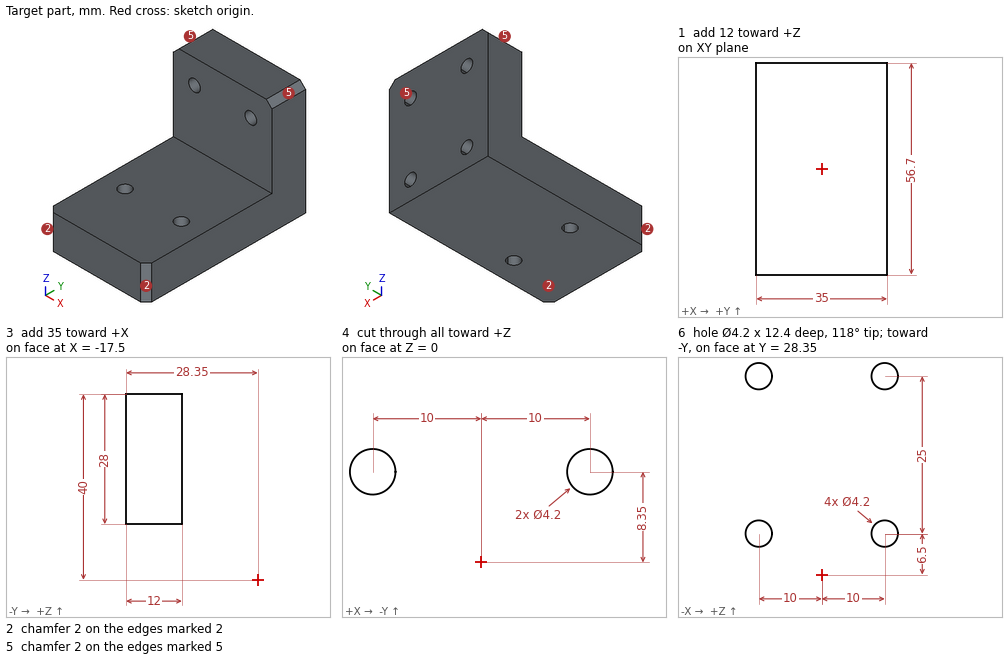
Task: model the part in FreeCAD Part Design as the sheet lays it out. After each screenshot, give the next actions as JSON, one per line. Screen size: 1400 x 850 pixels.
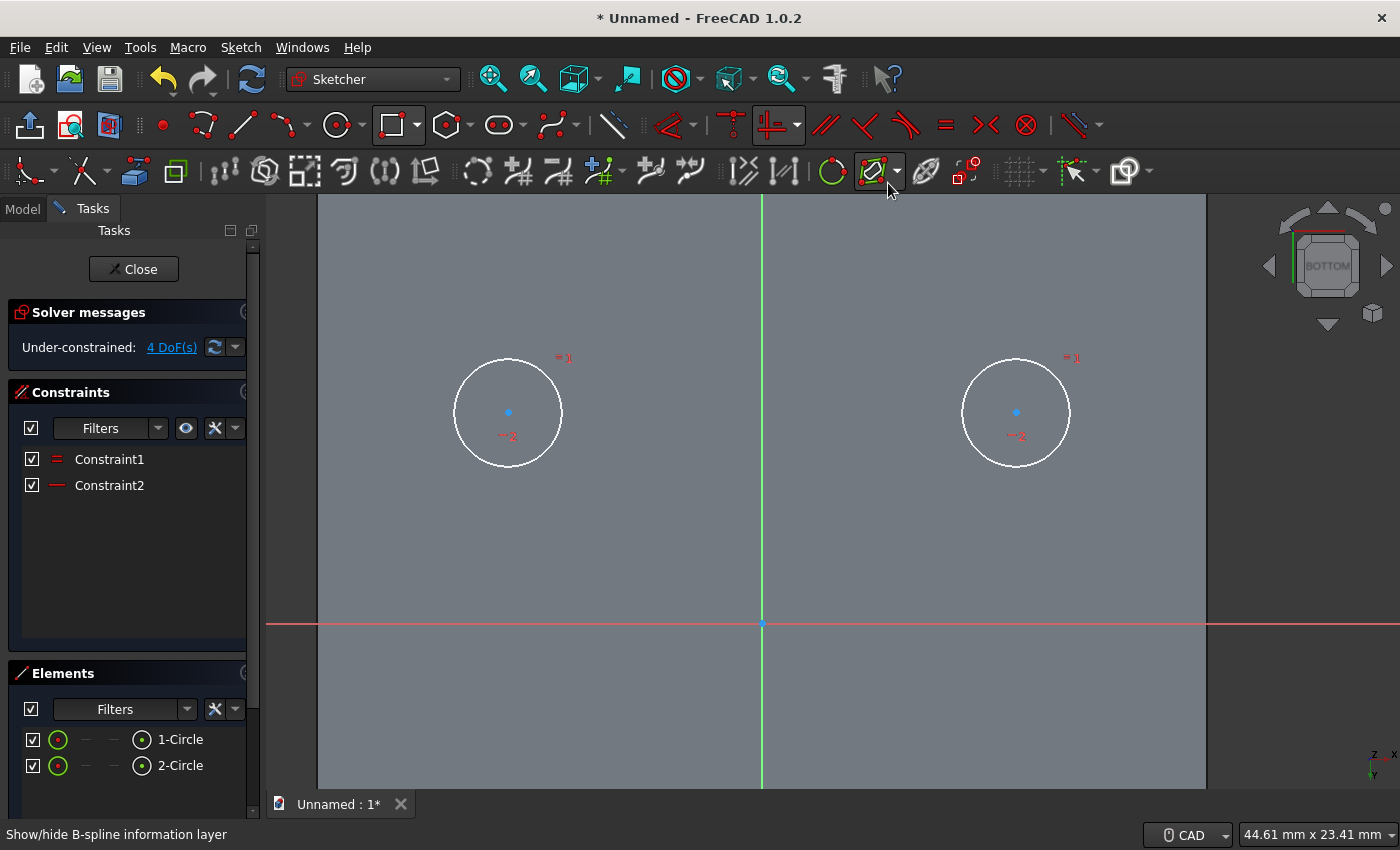
{"action": "left_click", "coordinate": [668, 126]}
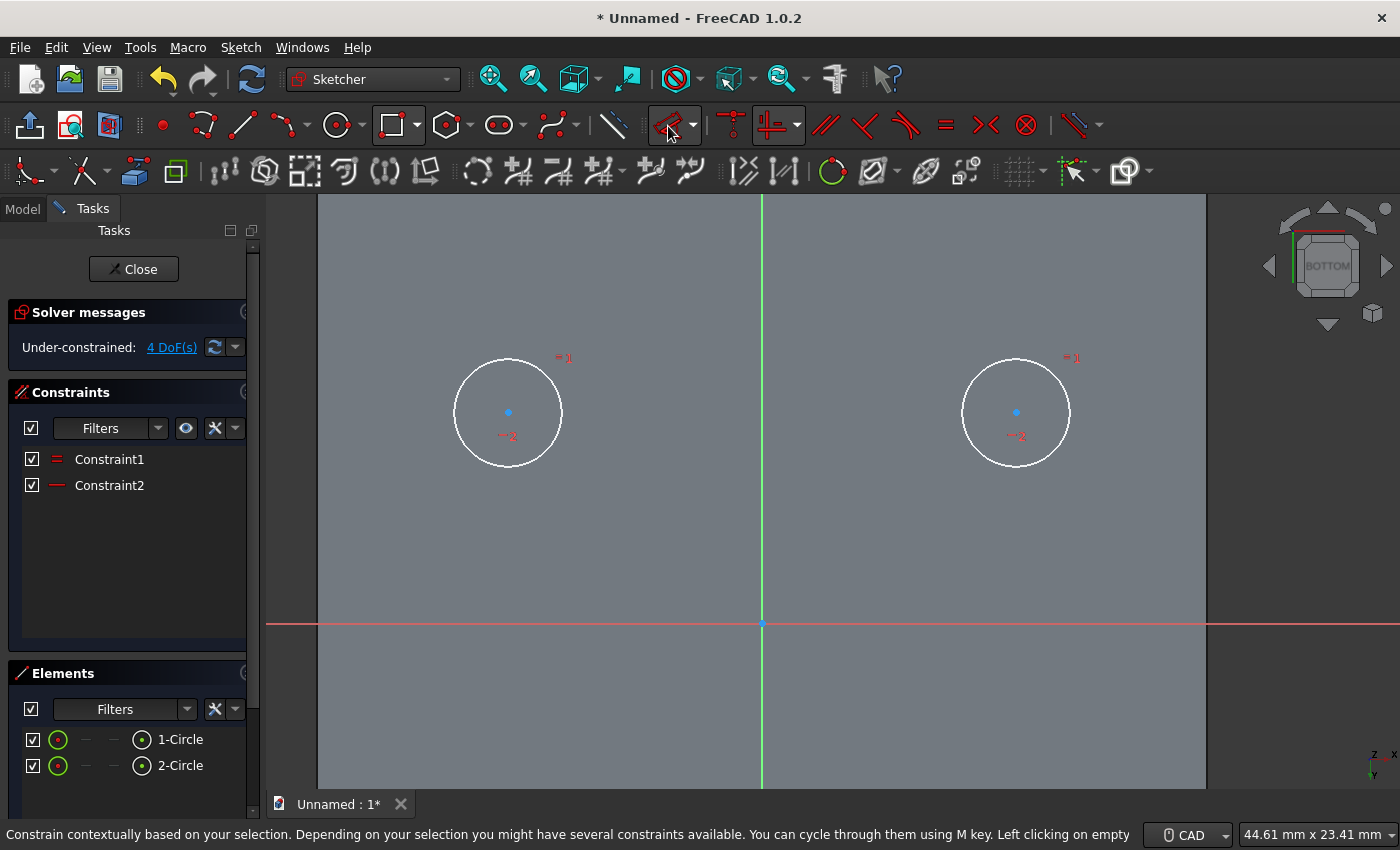
{"action": "left_click", "coordinate": [1054, 375]}
{"action": "left_click", "coordinate": [1077, 352]}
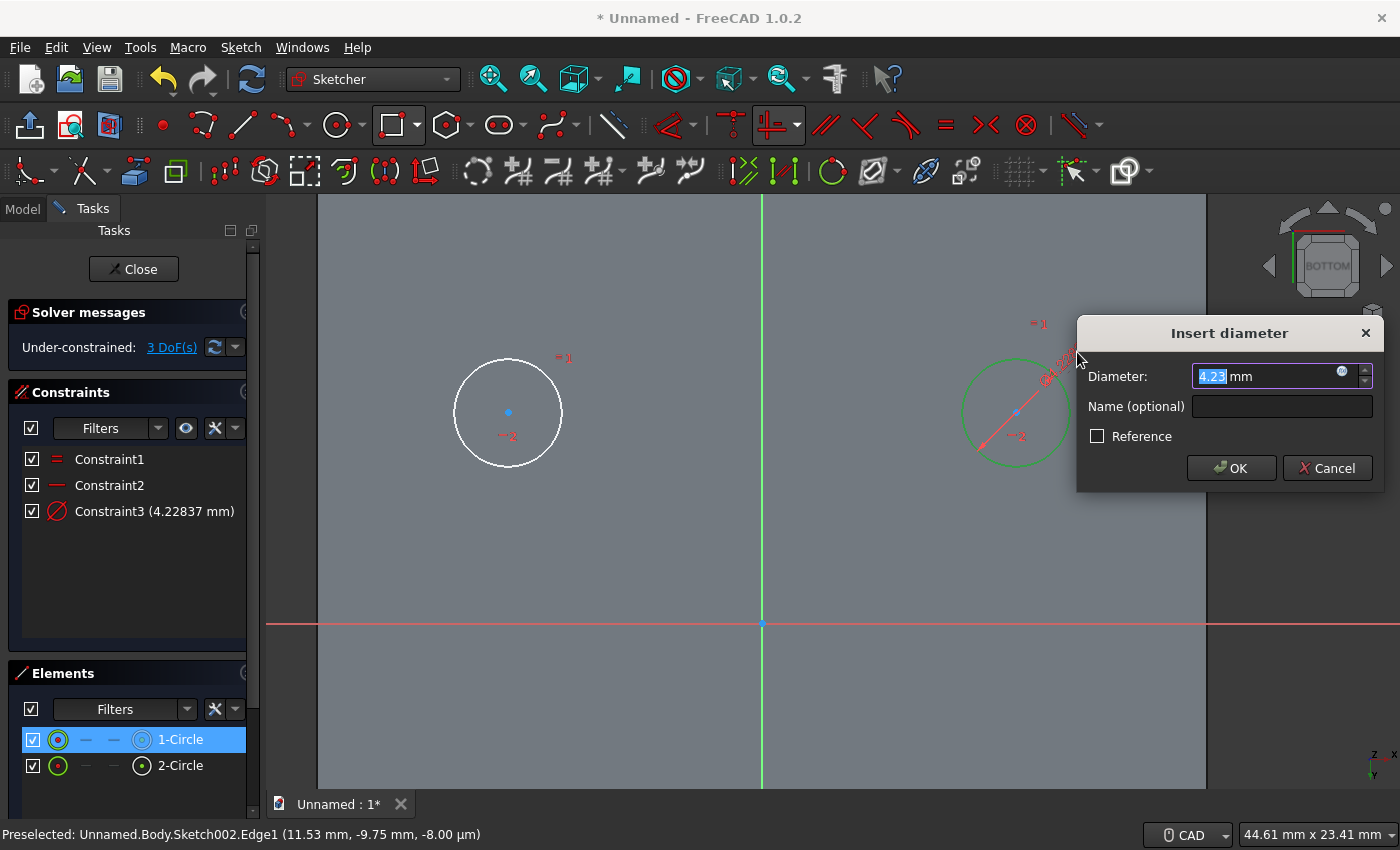
{"action": "type", "text": "4.2"}
{"action": "key", "text": "Return"}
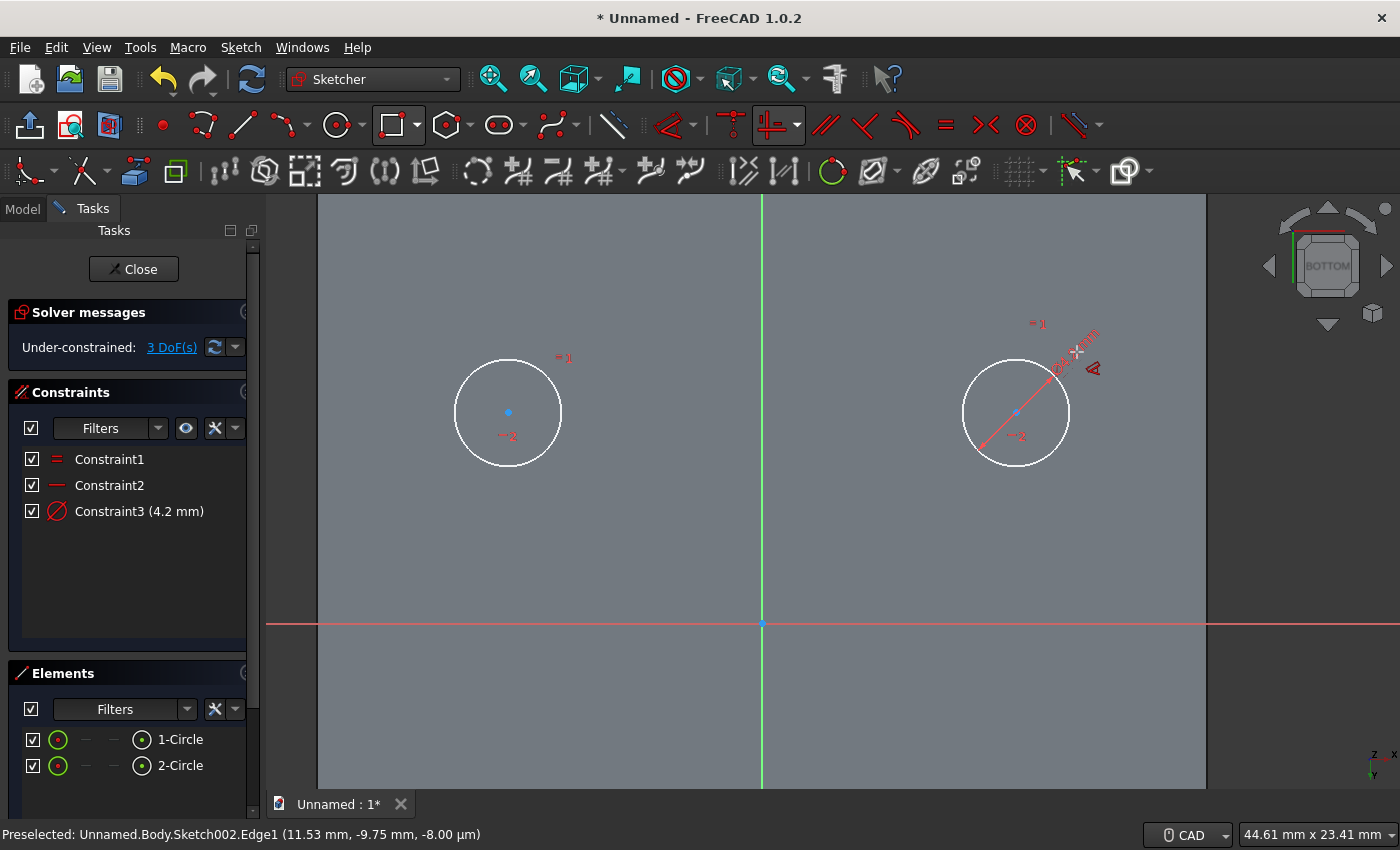
{"action": "left_click", "coordinate": [1016, 413]}
{"action": "left_click", "coordinate": [889, 658]}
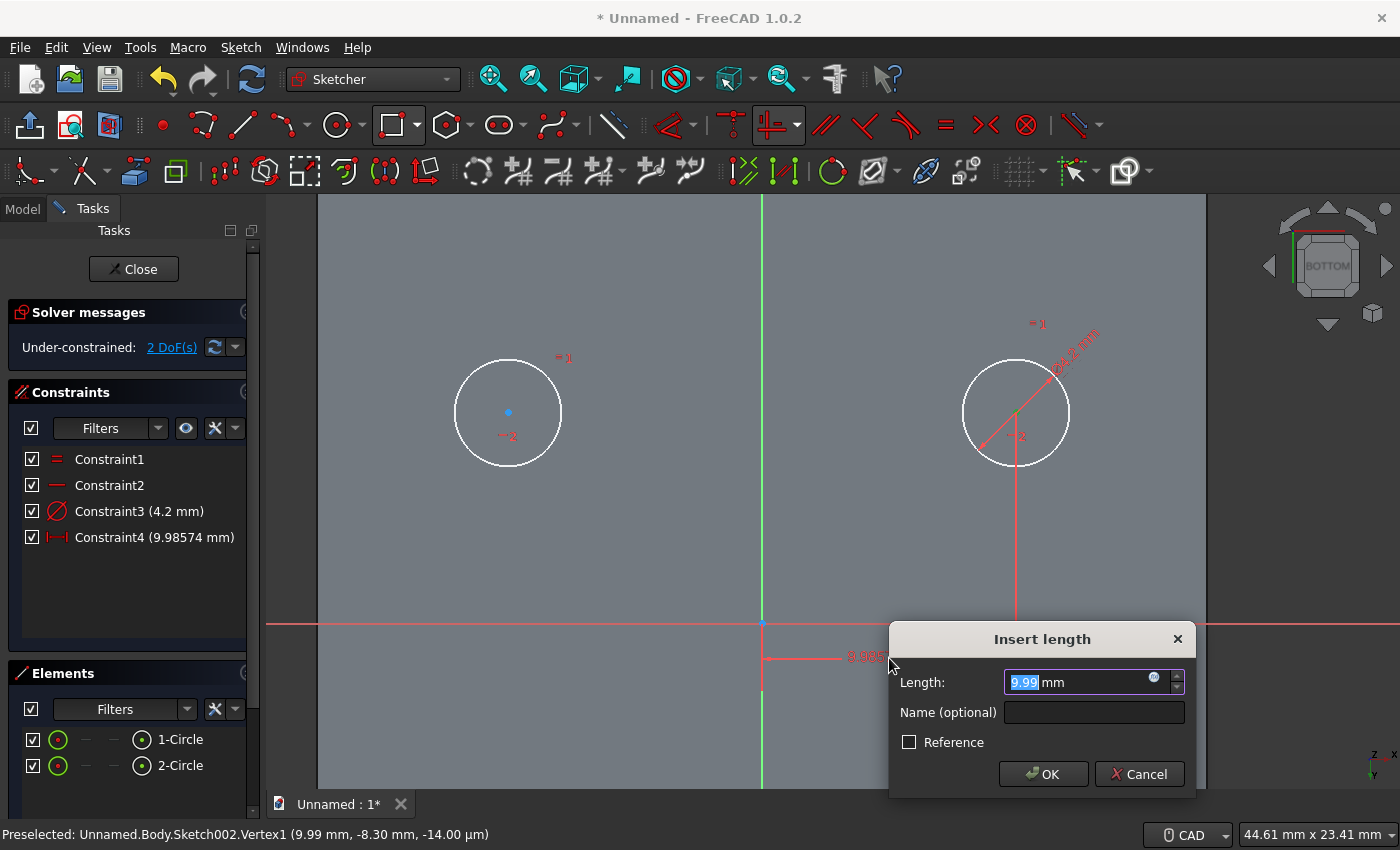
{"action": "type", "text": "10"}
{"action": "key", "text": "Return"}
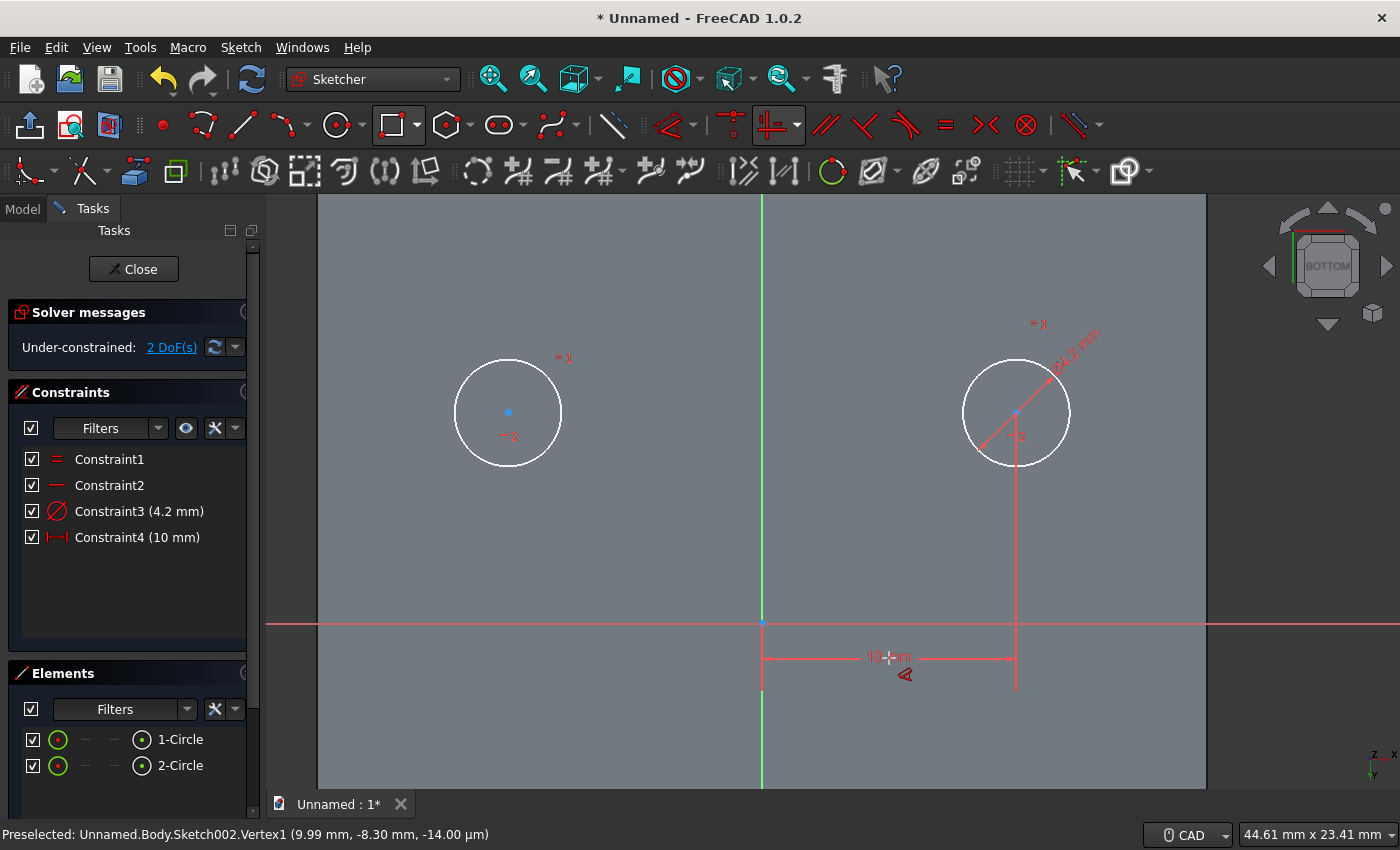
{"action": "left_click", "coordinate": [508, 413]}
{"action": "left_click", "coordinate": [635, 658]}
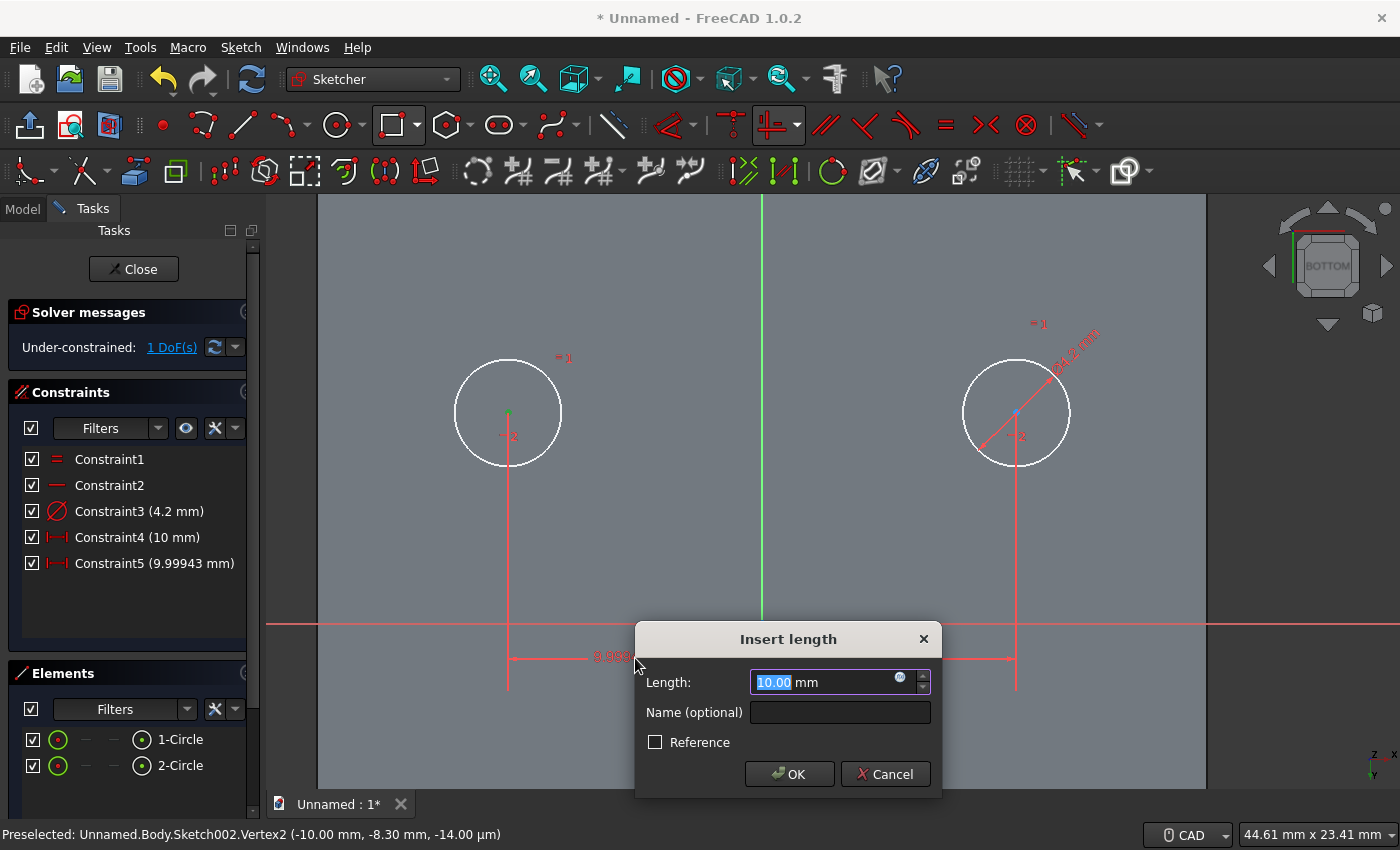
{"action": "type", "text": "10"}
{"action": "key", "text": "Return"}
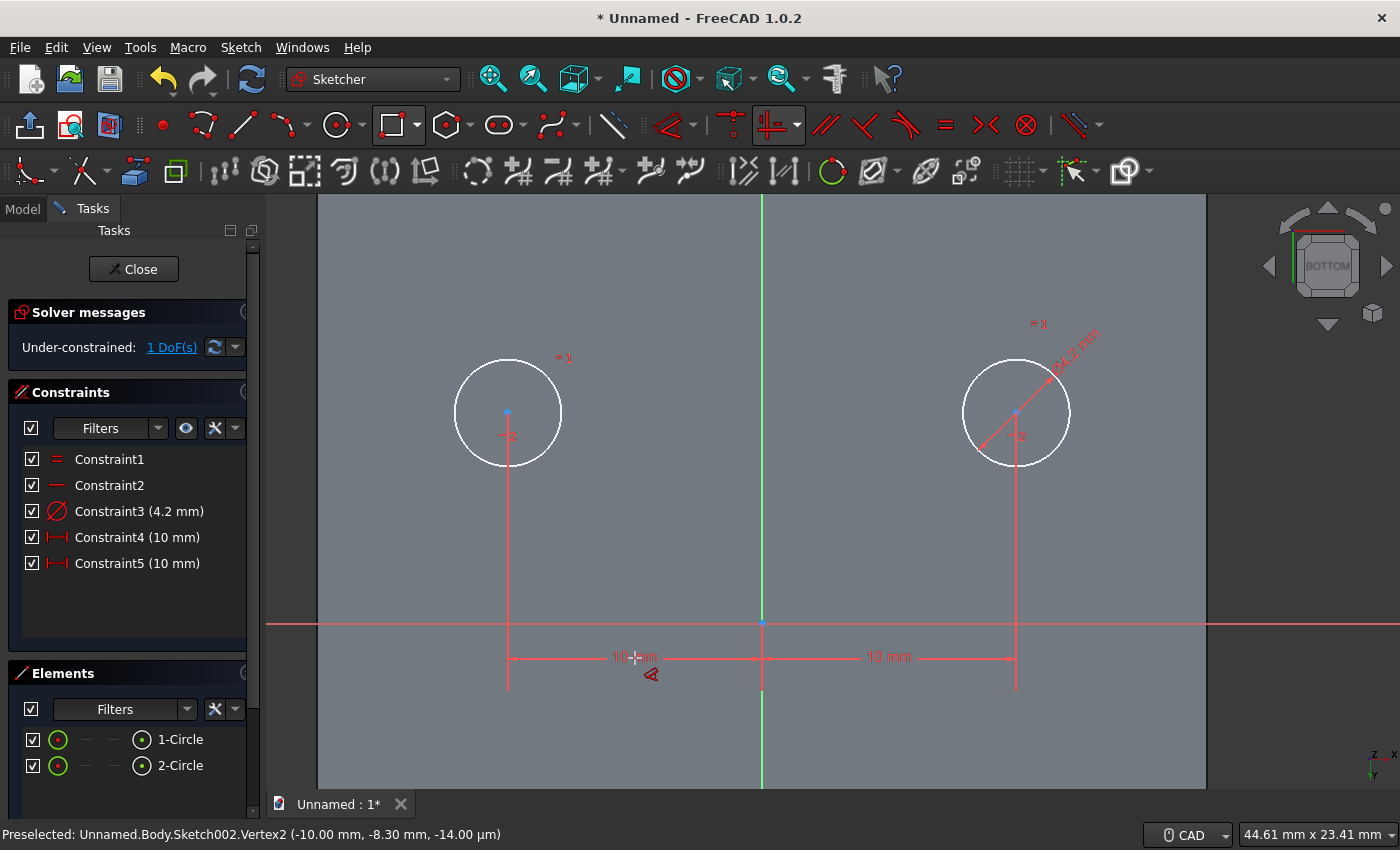
{"action": "left_click", "coordinate": [1016, 413]}
{"action": "left_click", "coordinate": [1050, 518]}